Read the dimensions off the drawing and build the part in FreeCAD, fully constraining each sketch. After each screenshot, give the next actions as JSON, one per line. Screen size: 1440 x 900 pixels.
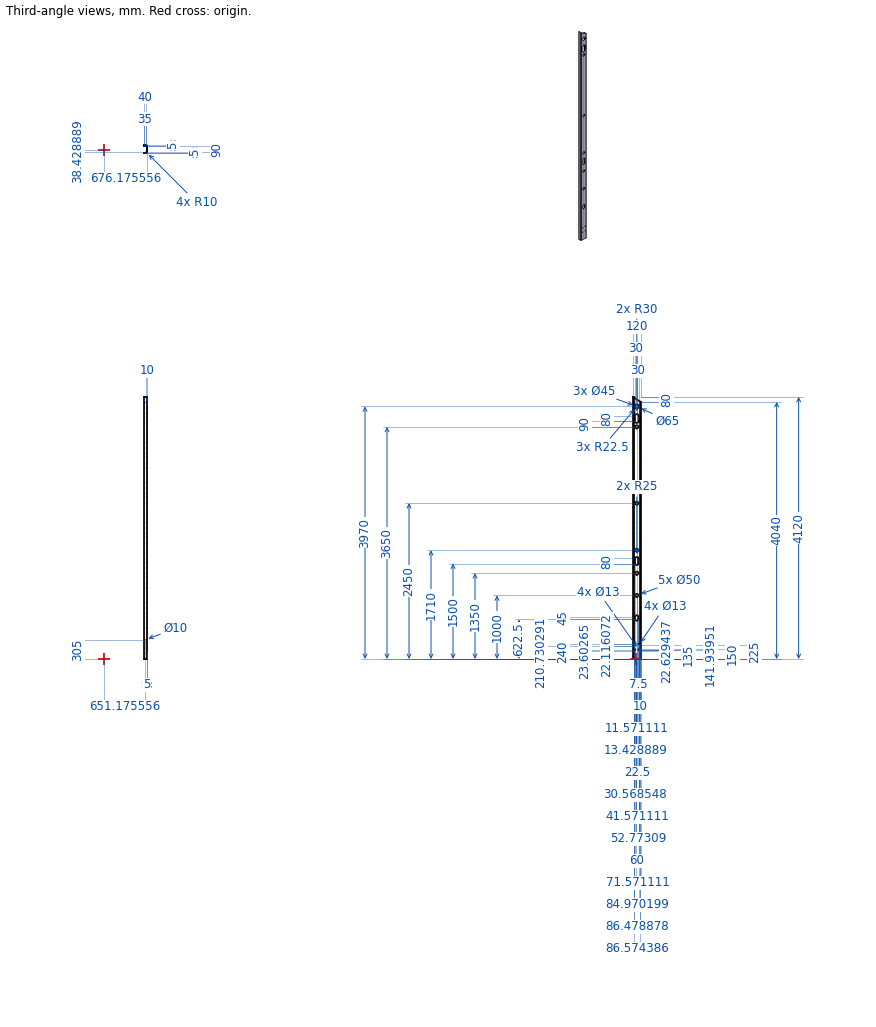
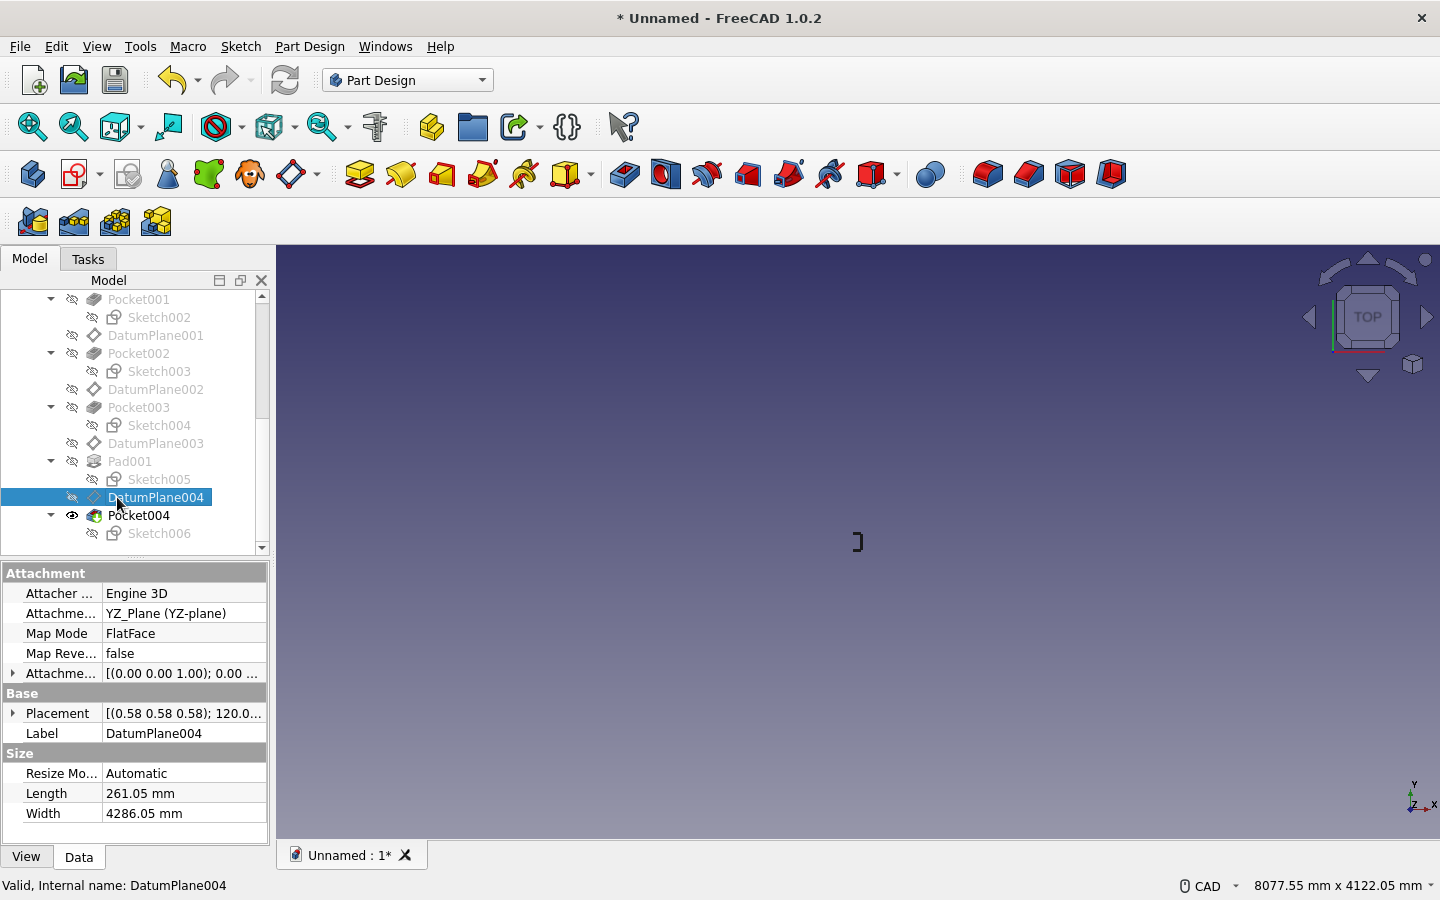
{"action": "key", "text": "v f"}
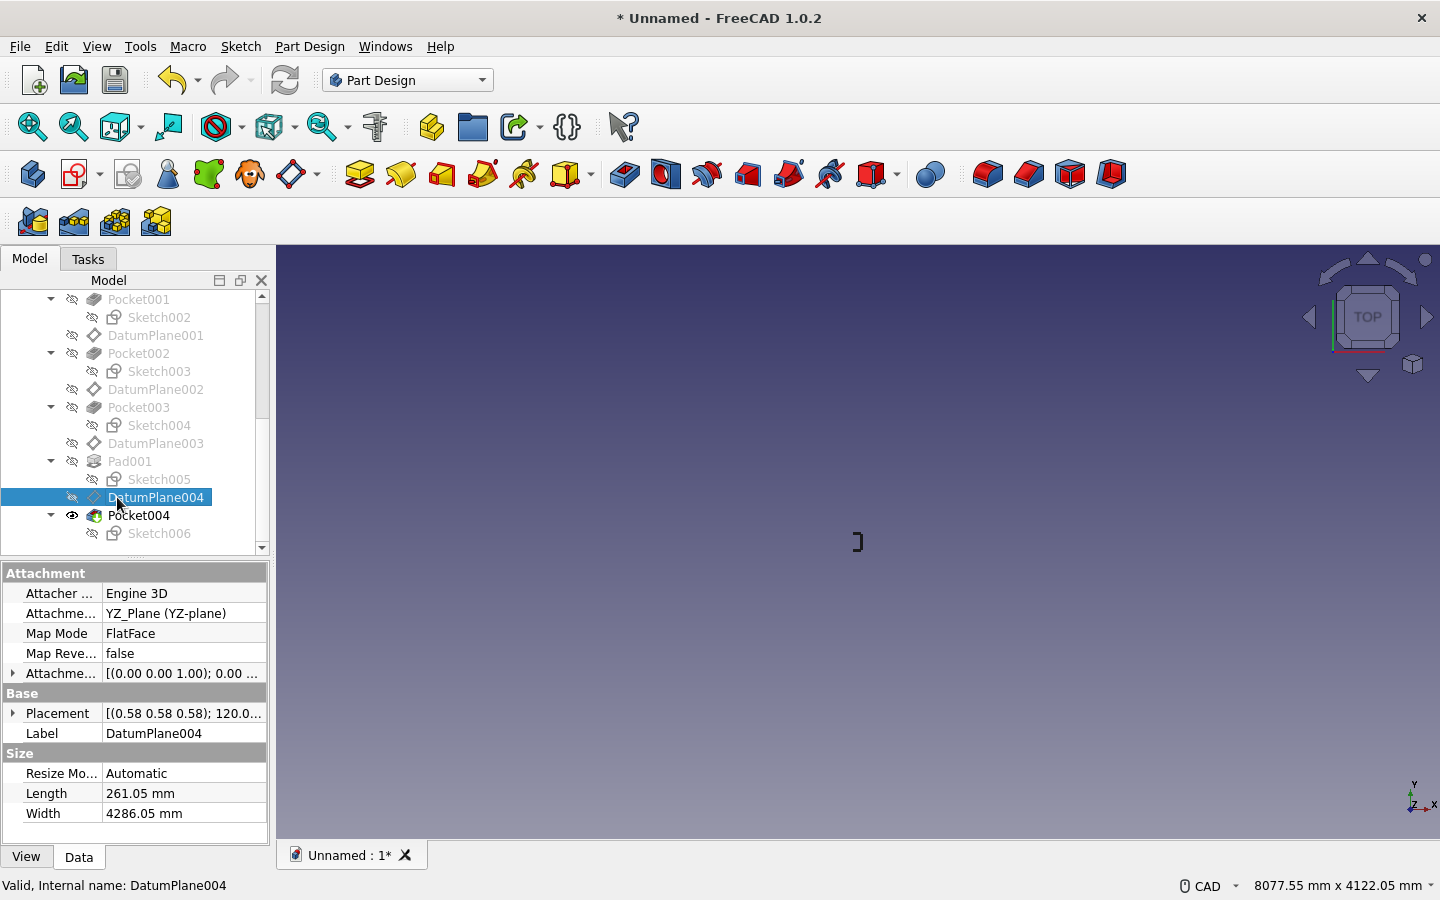
{"action": "scroll", "coordinate": [141, 421], "scroll_direction": "down", "scroll_amount": 3}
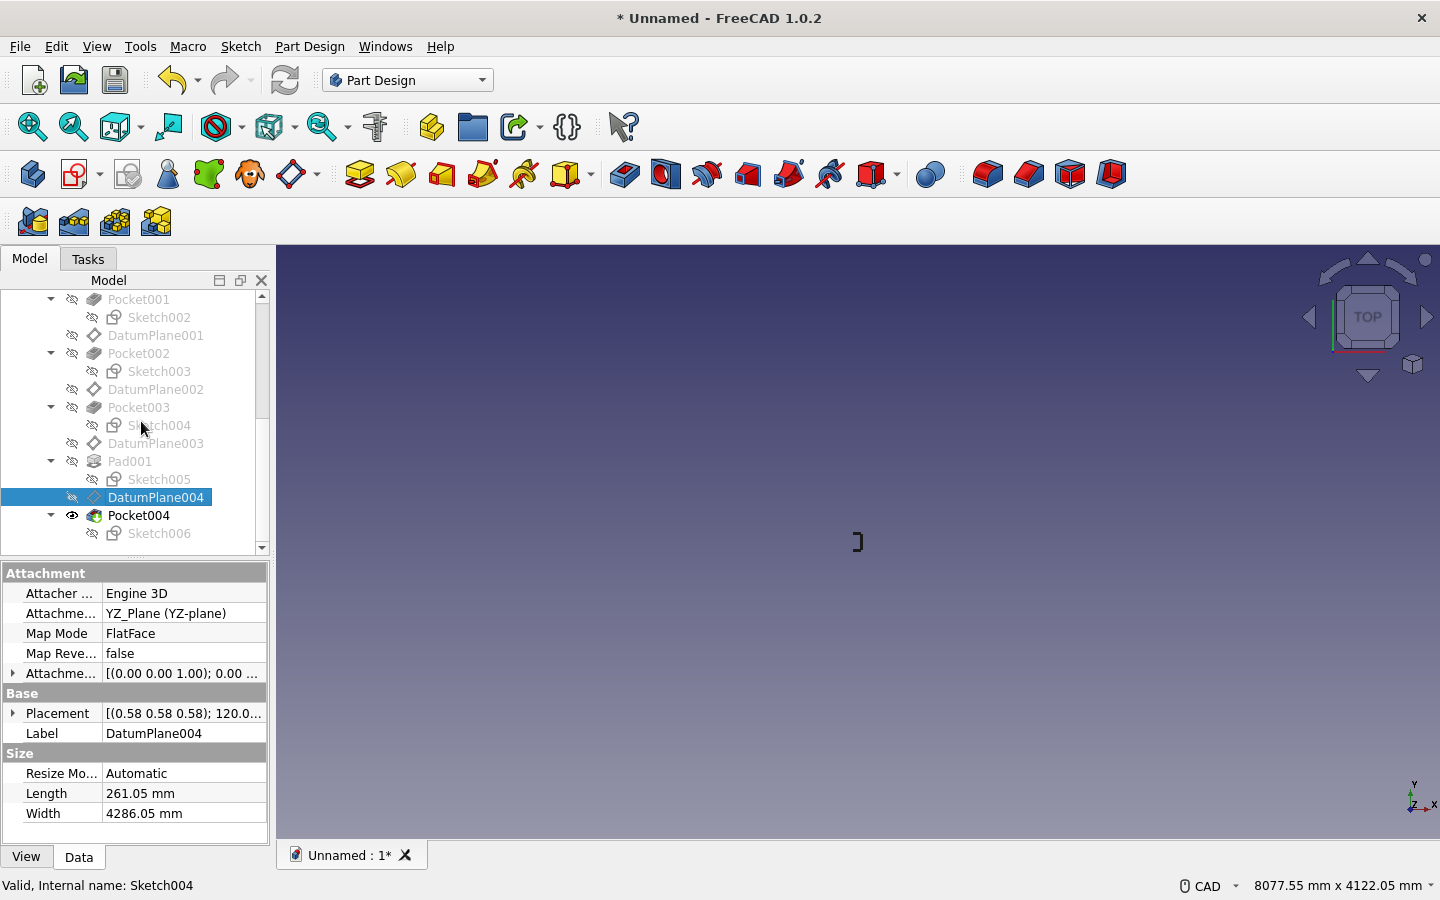
{"action": "scroll", "coordinate": [141, 421], "scroll_direction": "up", "scroll_amount": 15}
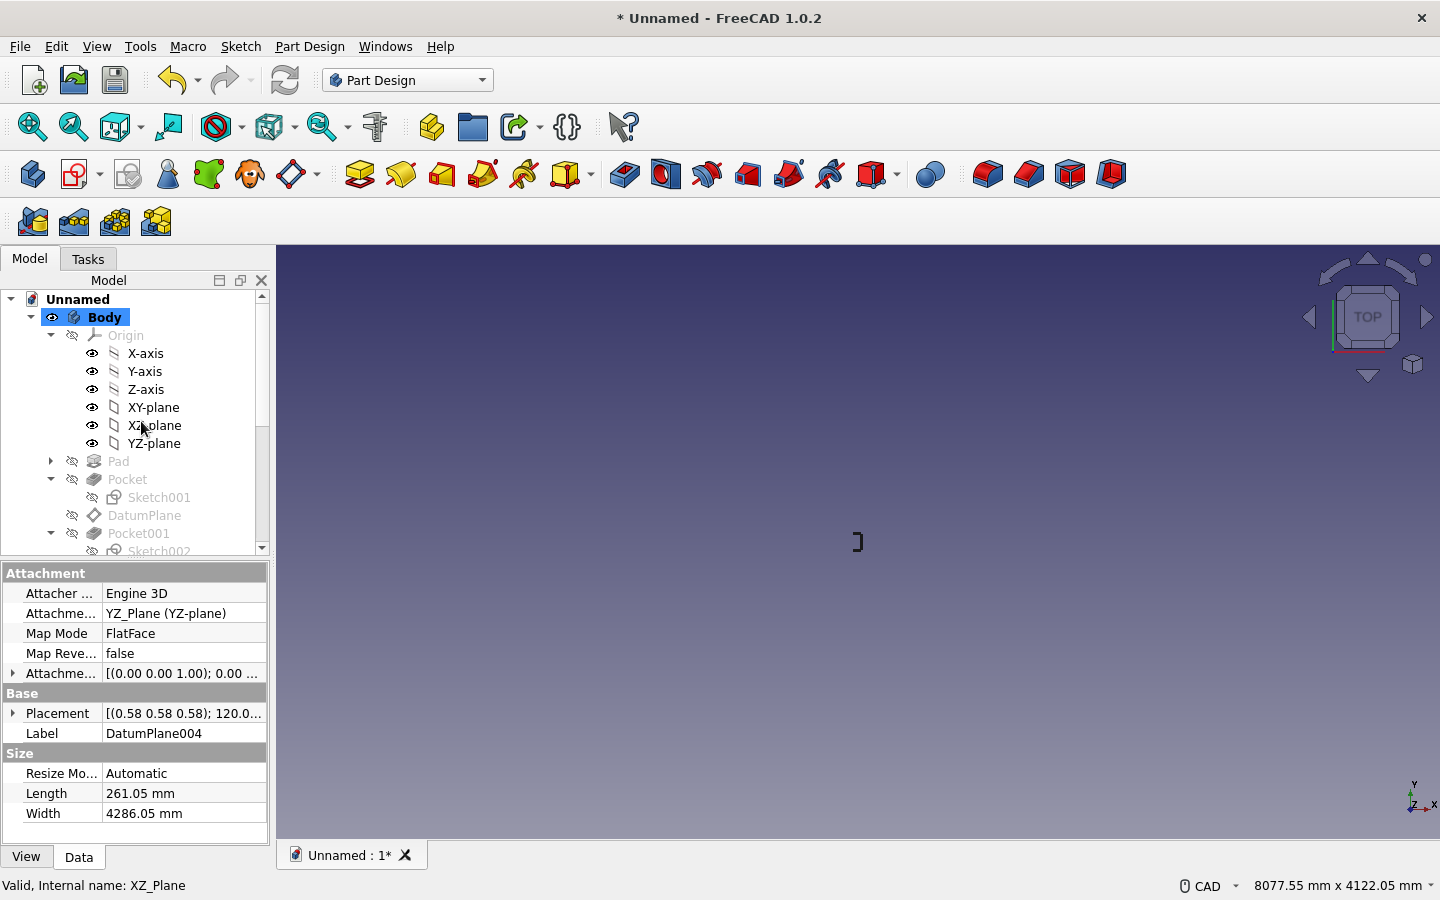
{"action": "left_click", "coordinate": [137, 443]}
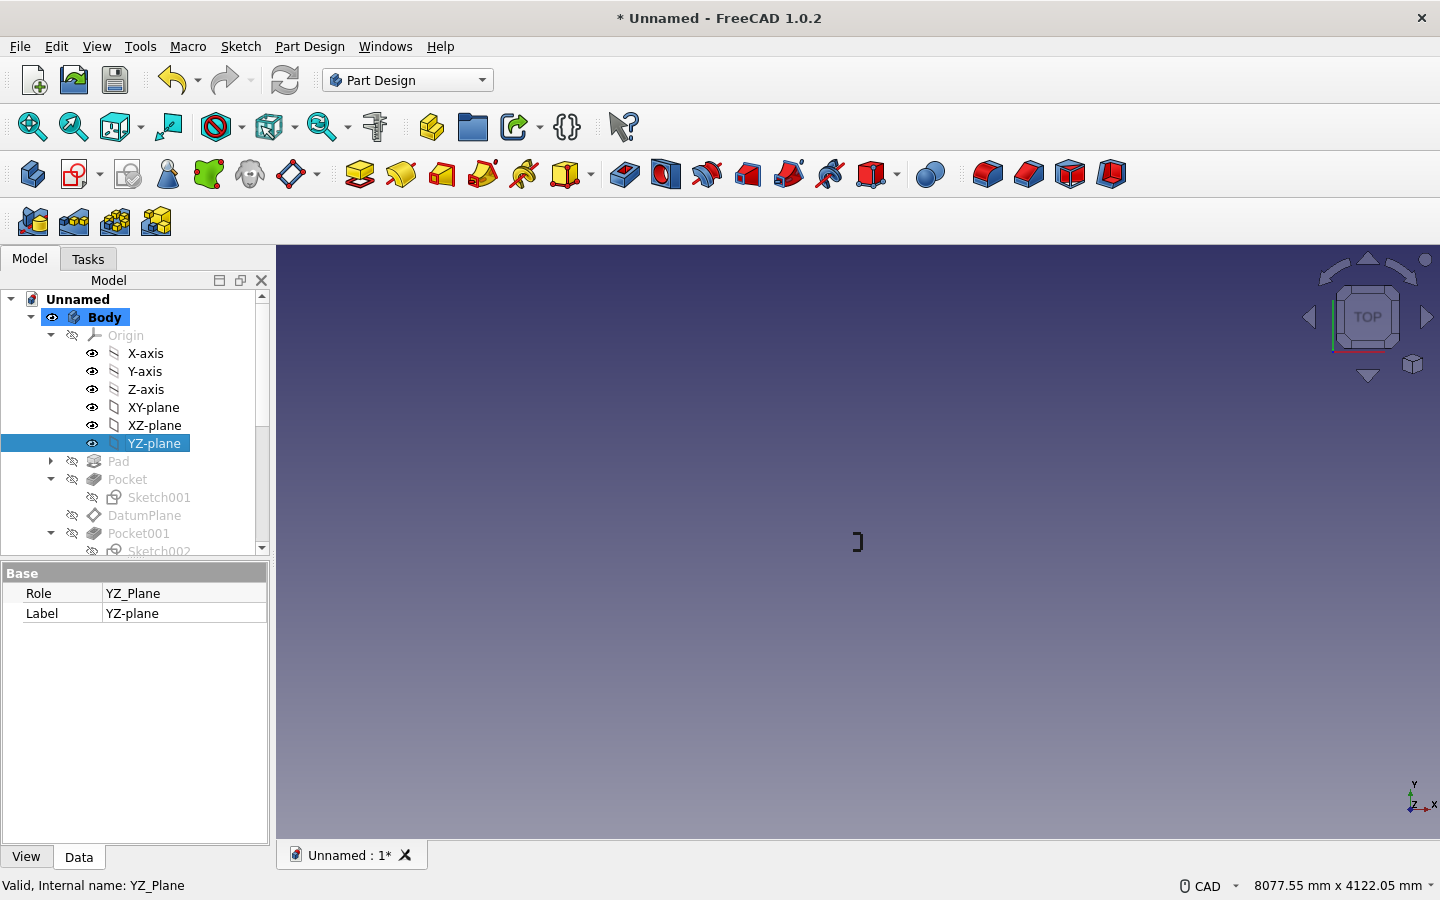
{"action": "left_click", "coordinate": [290, 174]}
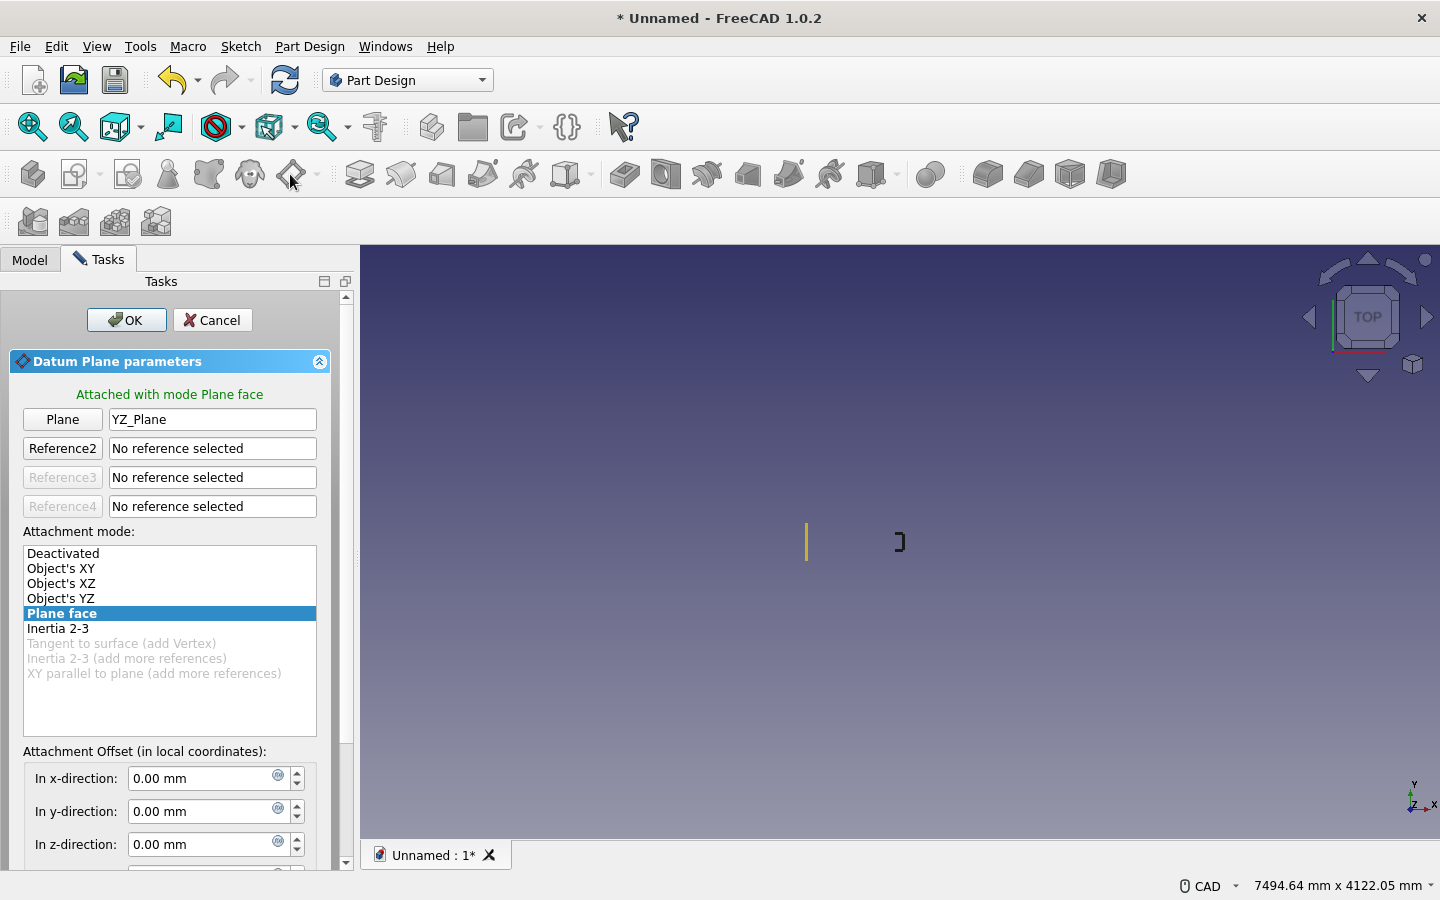
{"action": "triple_click", "coordinate": [210, 844]}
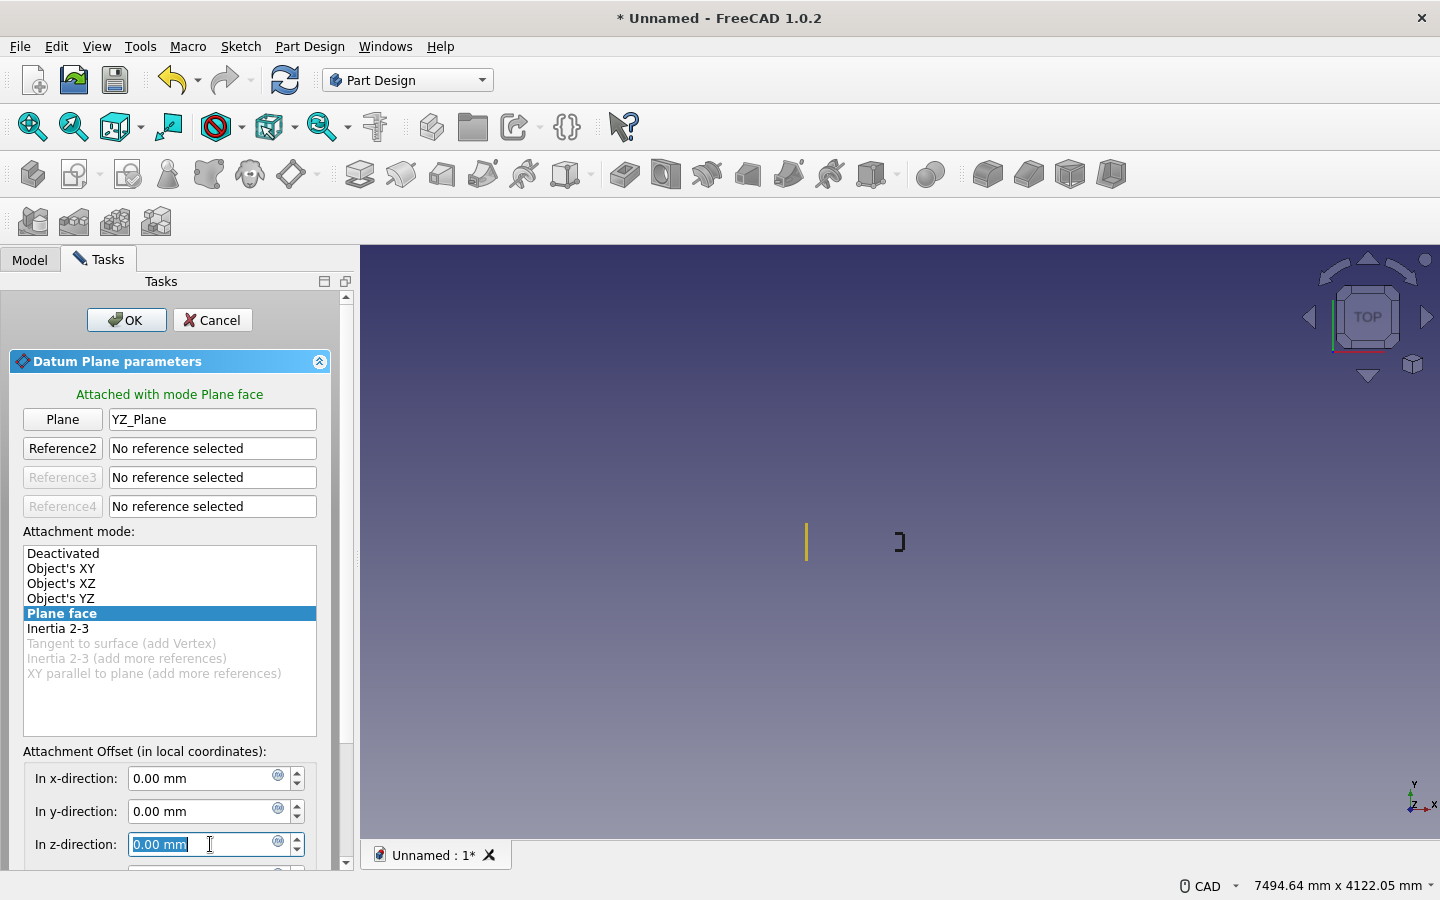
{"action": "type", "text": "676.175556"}
{"action": "key", "text": "Tab"}